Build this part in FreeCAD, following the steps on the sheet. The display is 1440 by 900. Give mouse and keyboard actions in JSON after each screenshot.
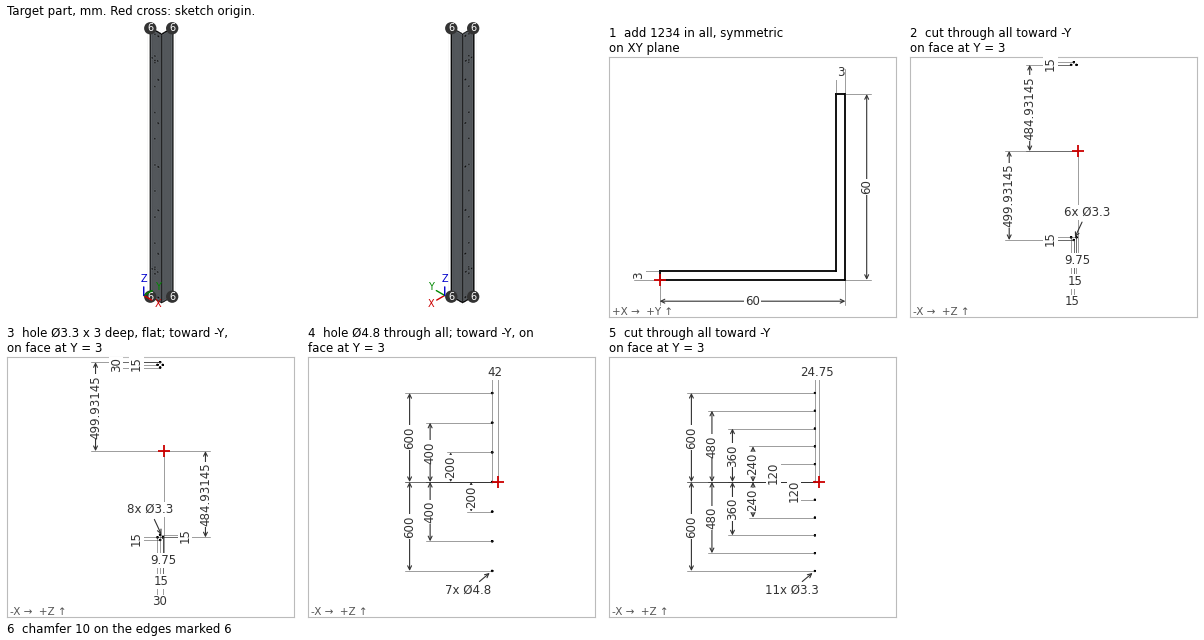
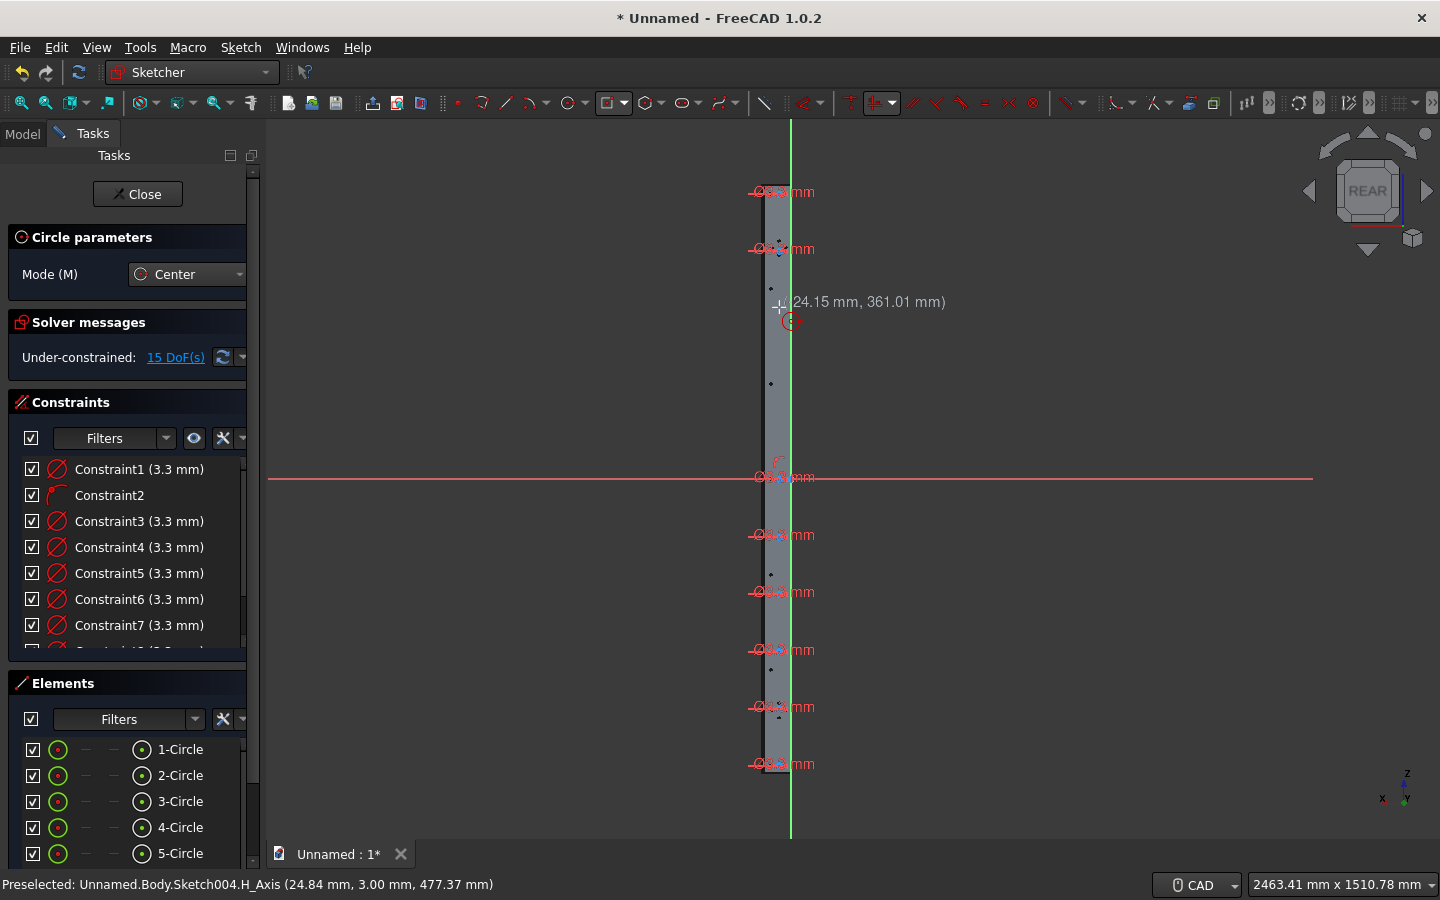
{"action": "scroll", "coordinate": [779, 308], "scroll_direction": "up", "scroll_amount": 2}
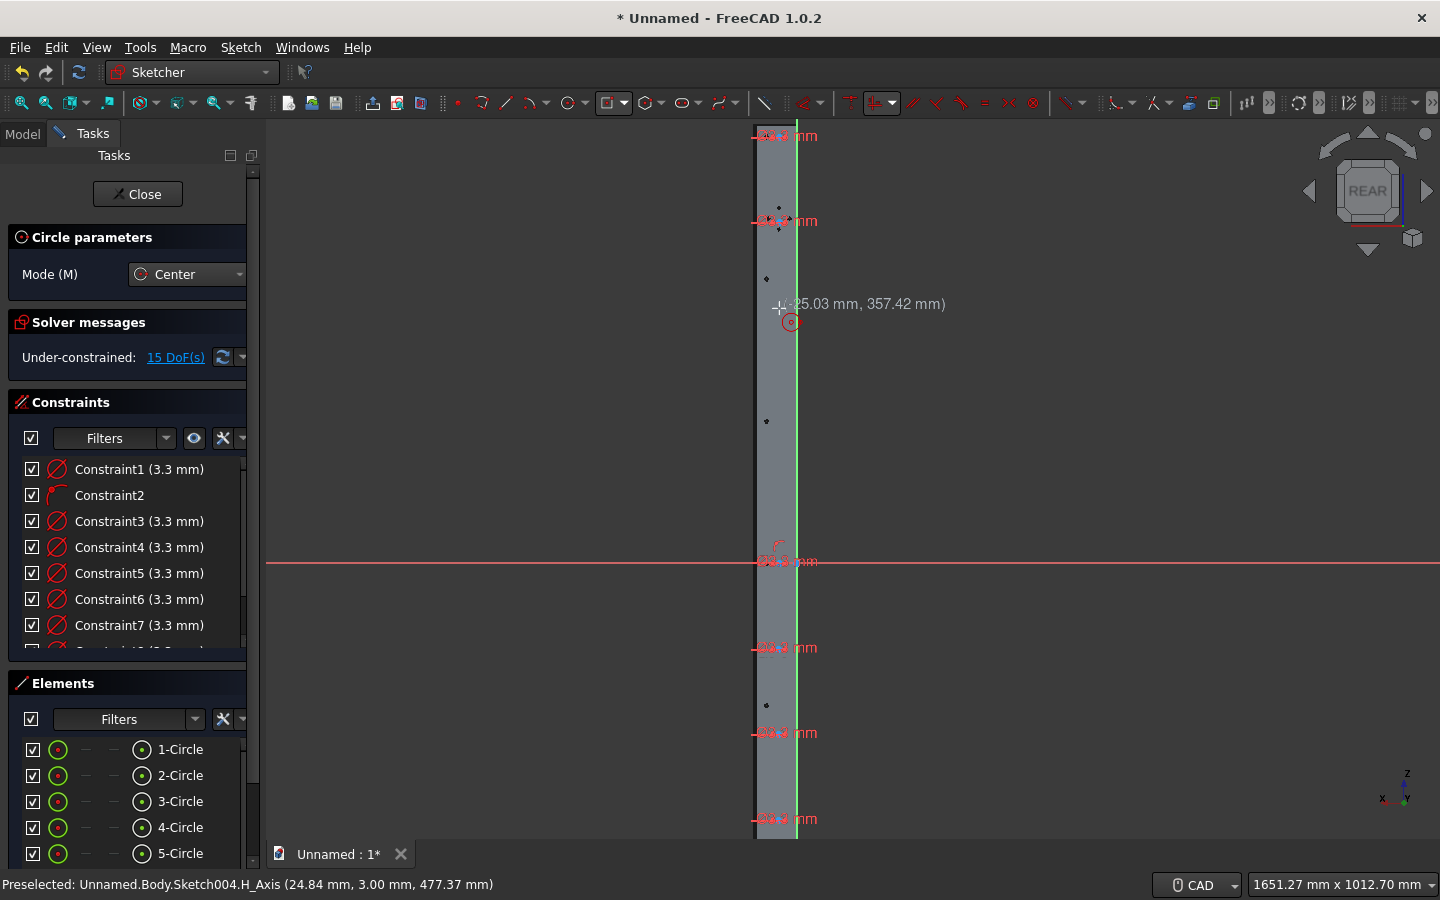
{"action": "left_click", "coordinate": [779, 308]}
{"action": "mouse_move", "coordinate": [780, 307]}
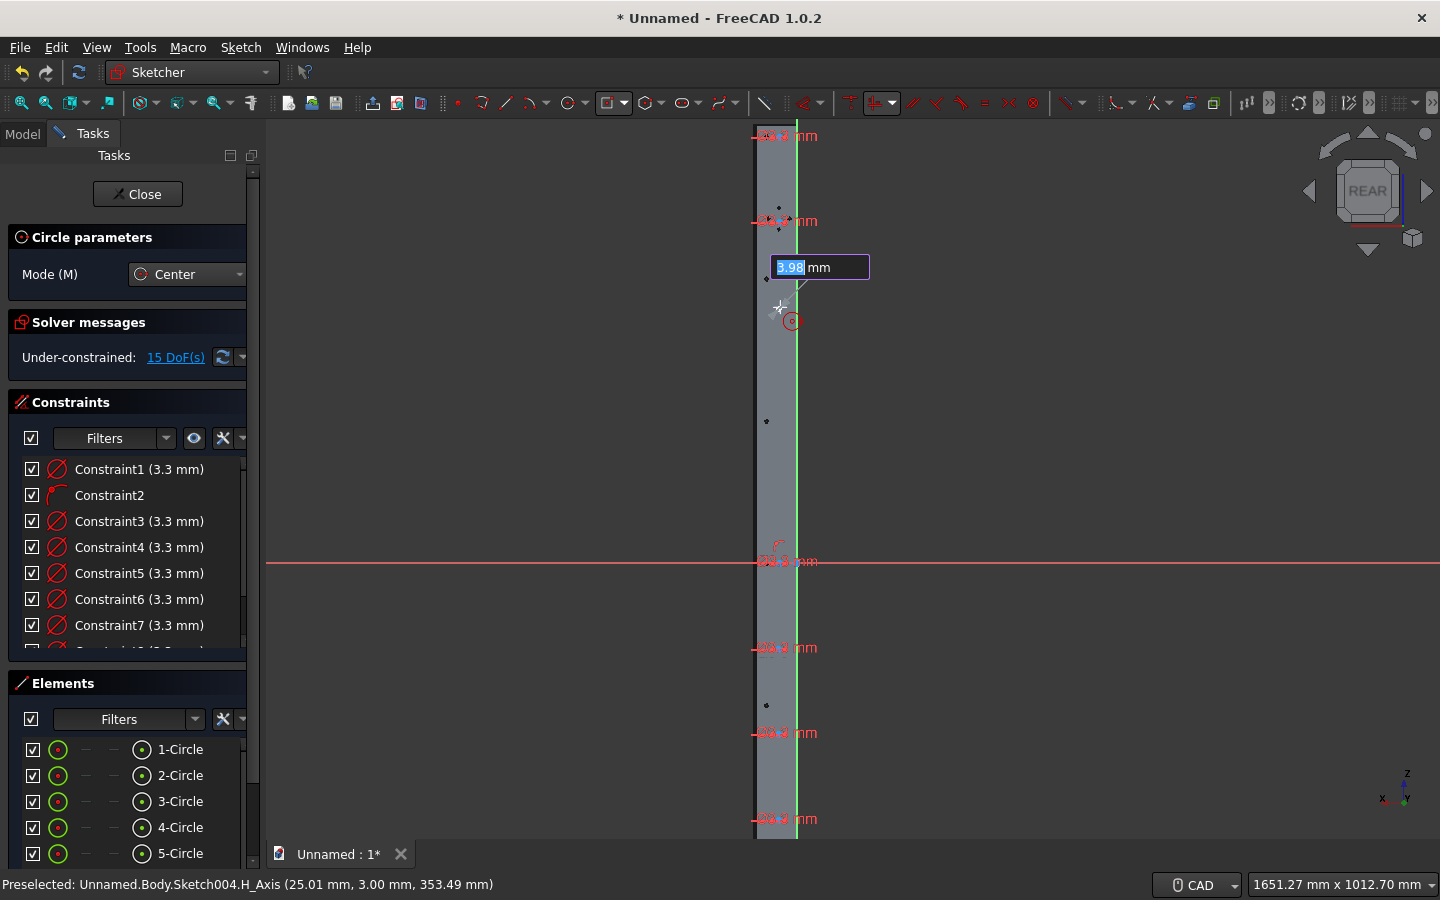
{"action": "type", "text": "3.3"}
{"action": "key", "text": "Return"}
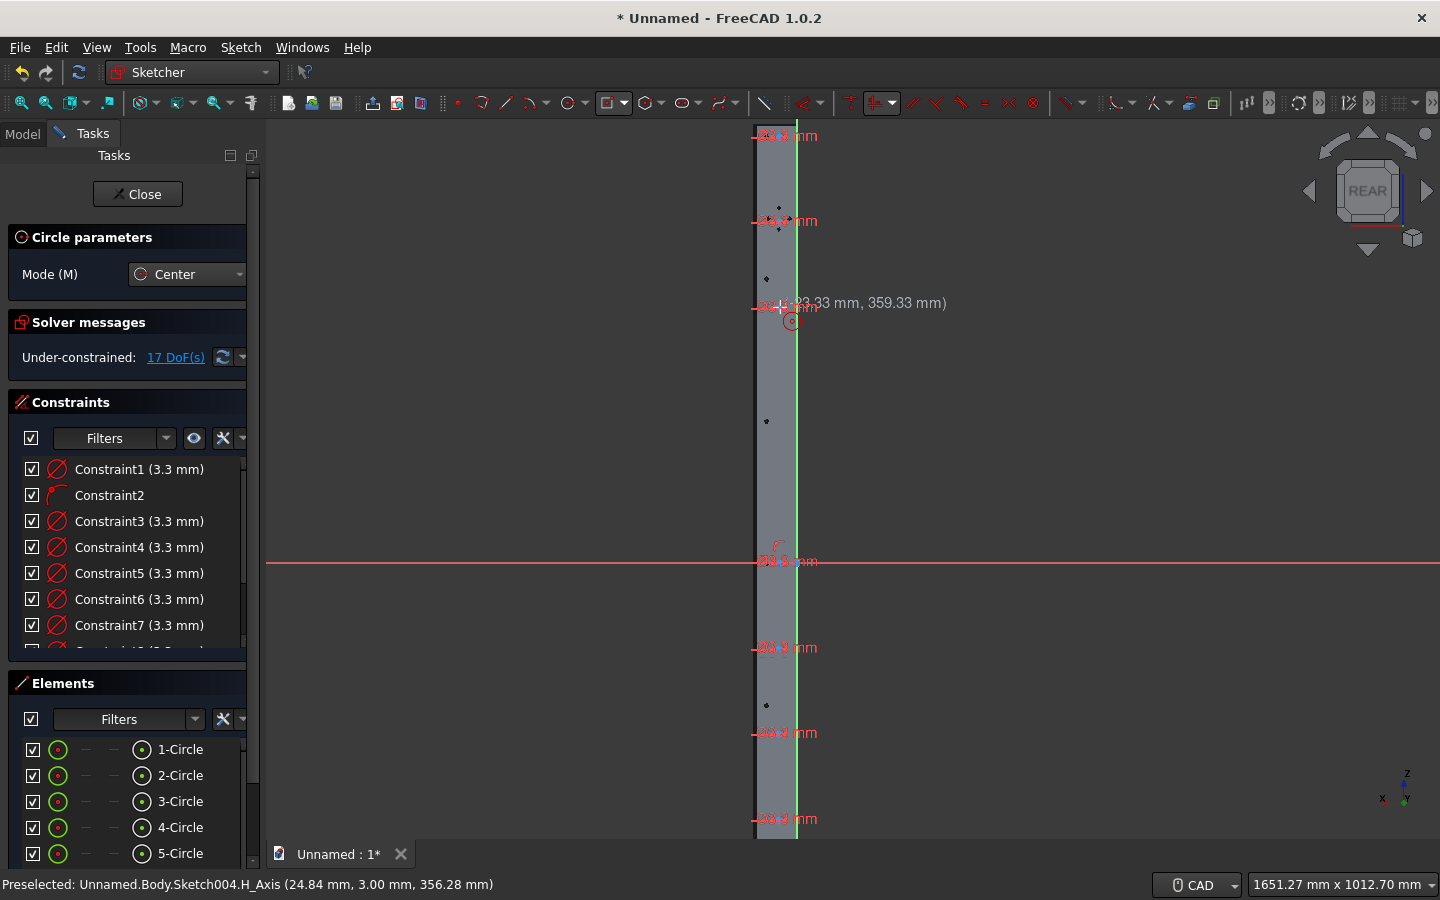
{"action": "scroll", "coordinate": [779, 393], "scroll_direction": "up", "scroll_amount": 15}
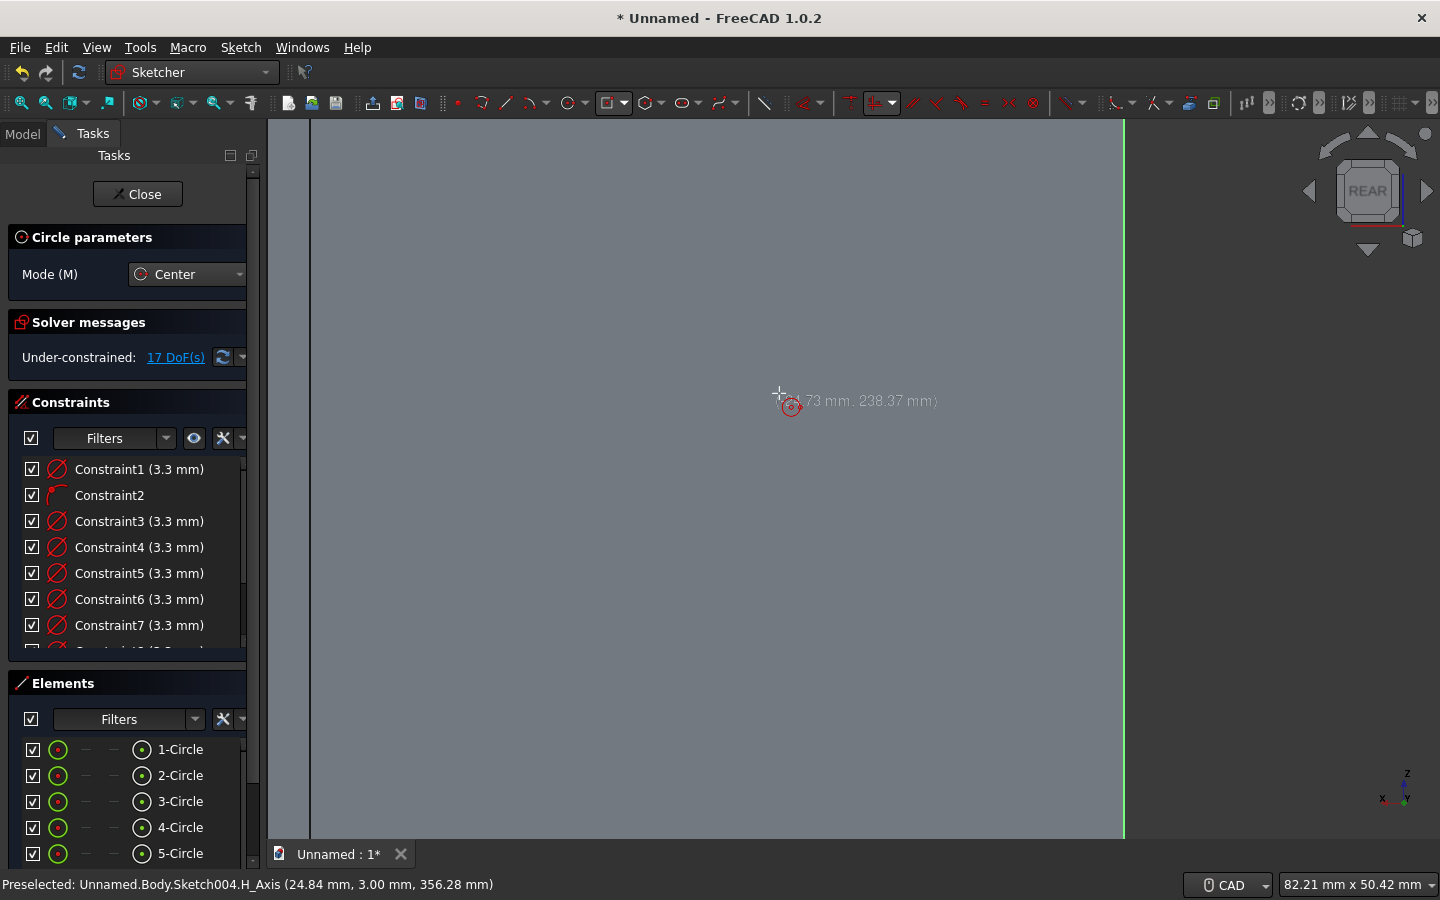
{"action": "scroll", "coordinate": [779, 364], "scroll_direction": "down", "scroll_amount": 17}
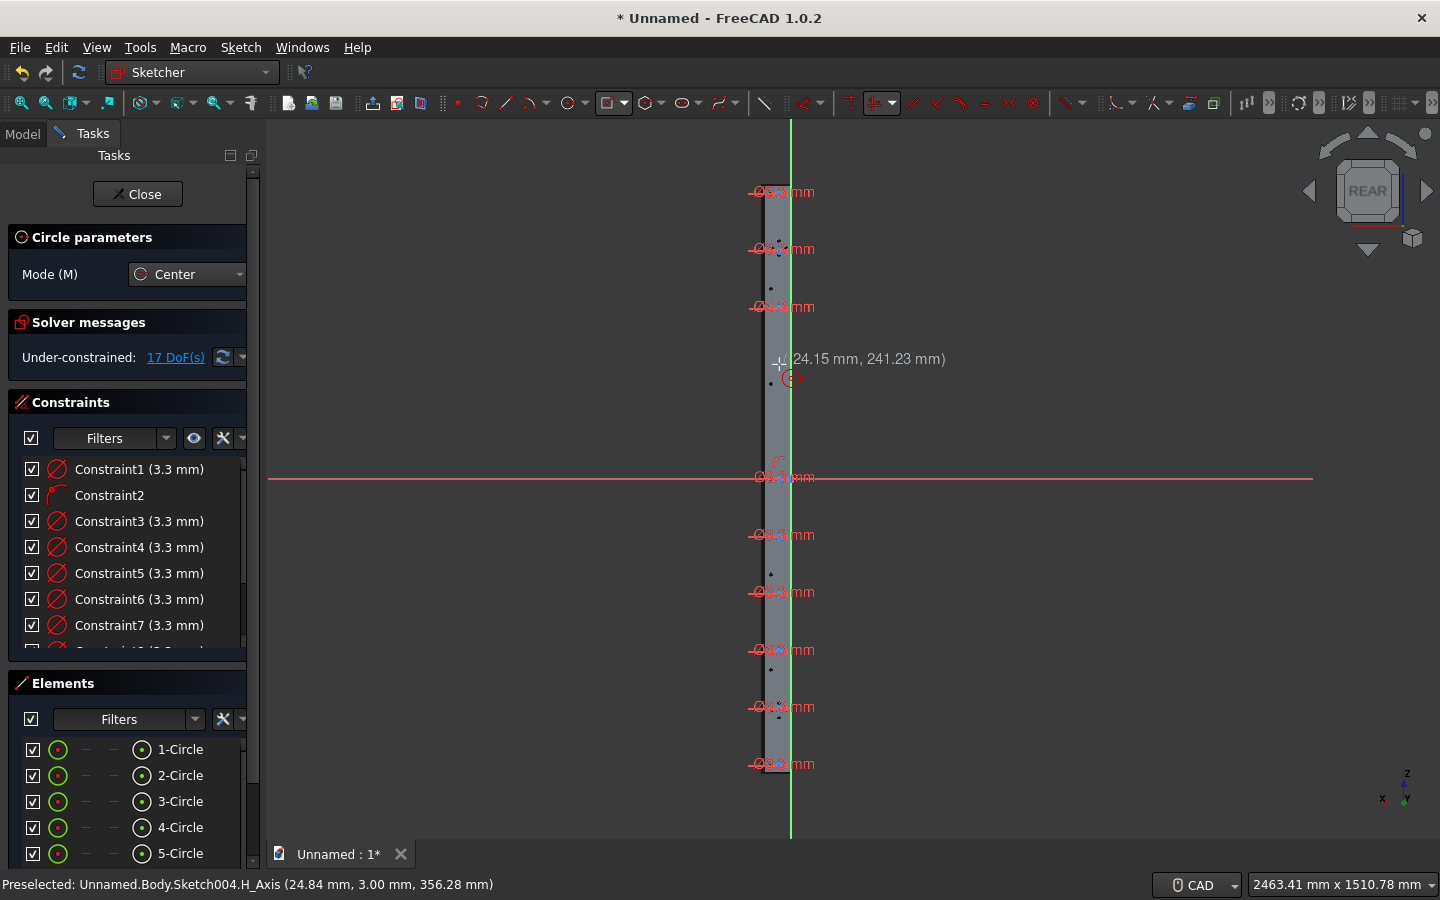
{"action": "scroll", "coordinate": [779, 365], "scroll_direction": "up", "scroll_amount": 2}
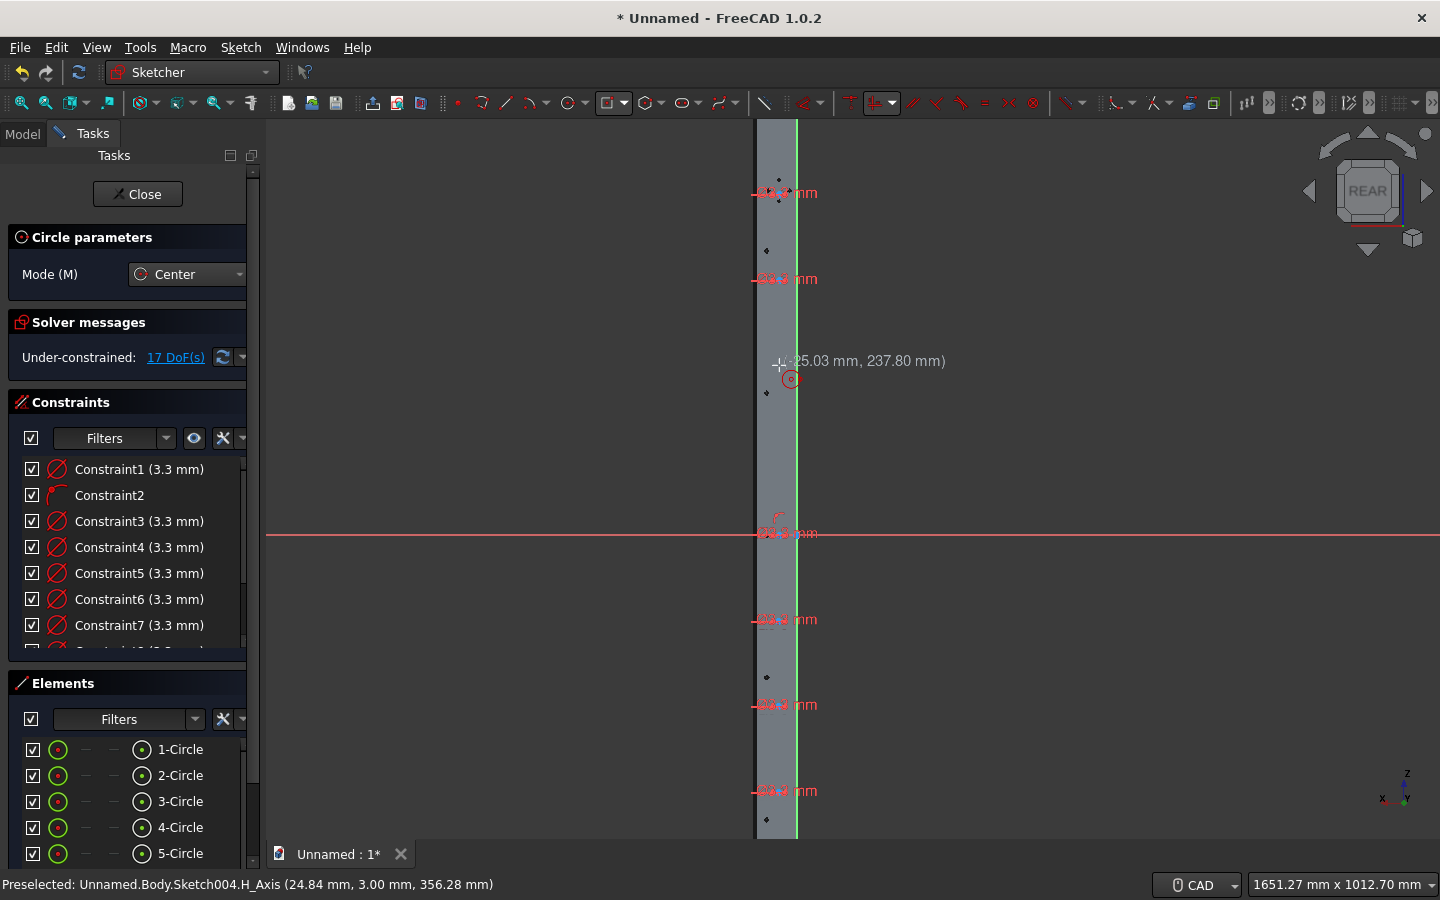
{"action": "left_click", "coordinate": [779, 365]}
{"action": "mouse_move", "coordinate": [780, 364]}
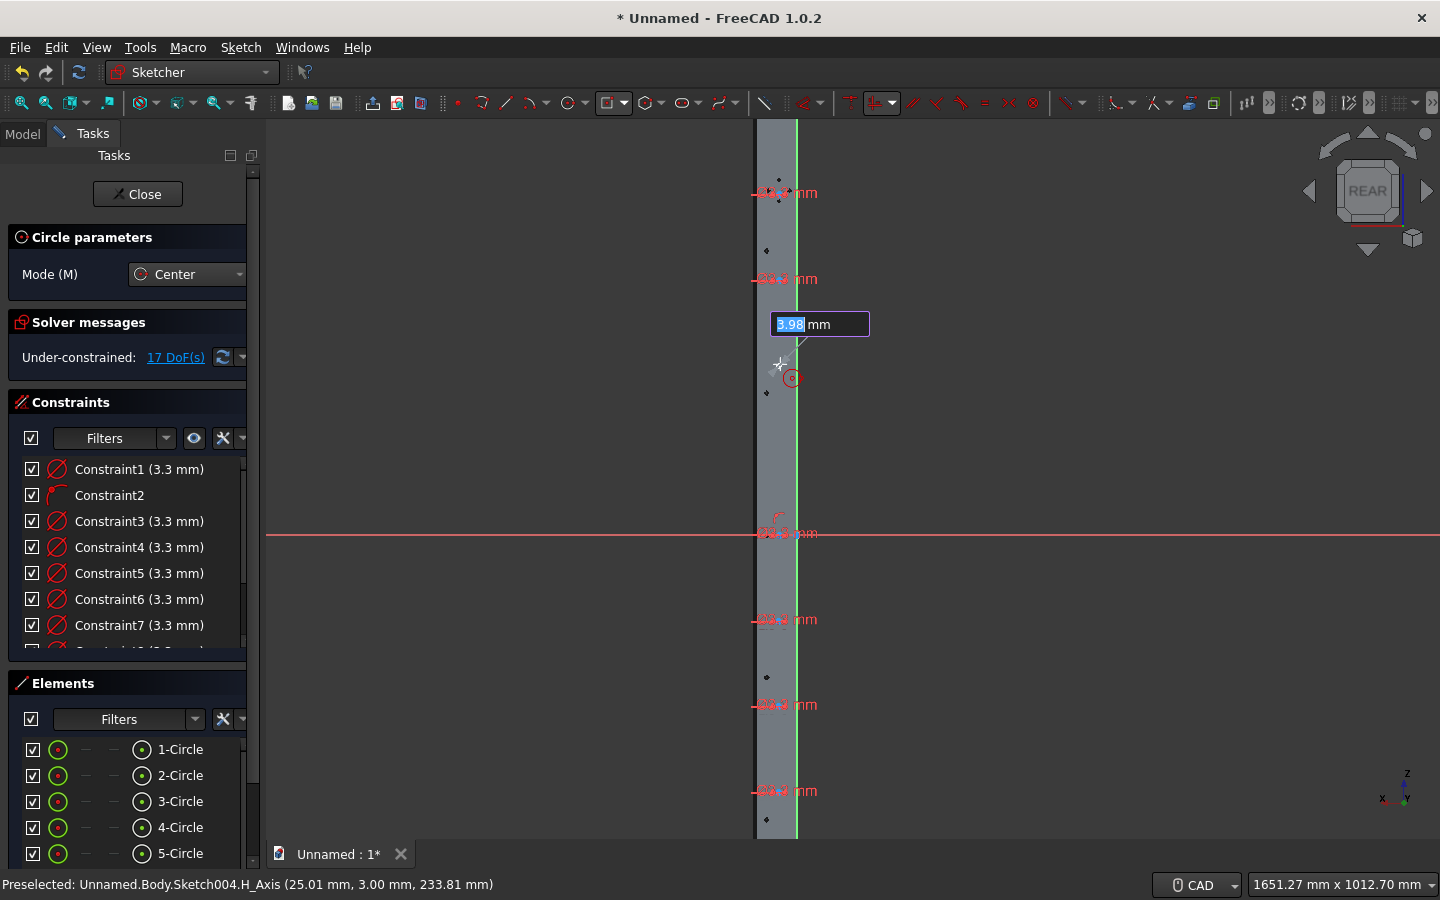
{"action": "type", "text": "3.3"}
{"action": "key", "text": "Return"}